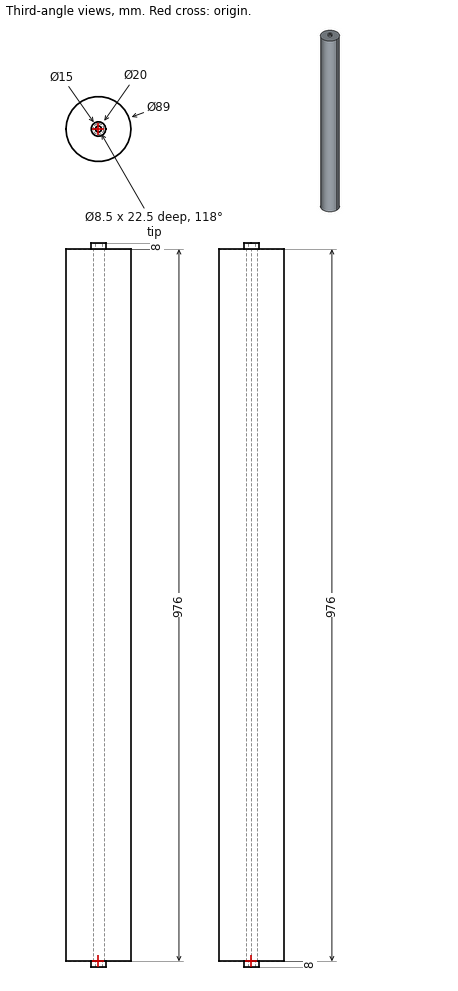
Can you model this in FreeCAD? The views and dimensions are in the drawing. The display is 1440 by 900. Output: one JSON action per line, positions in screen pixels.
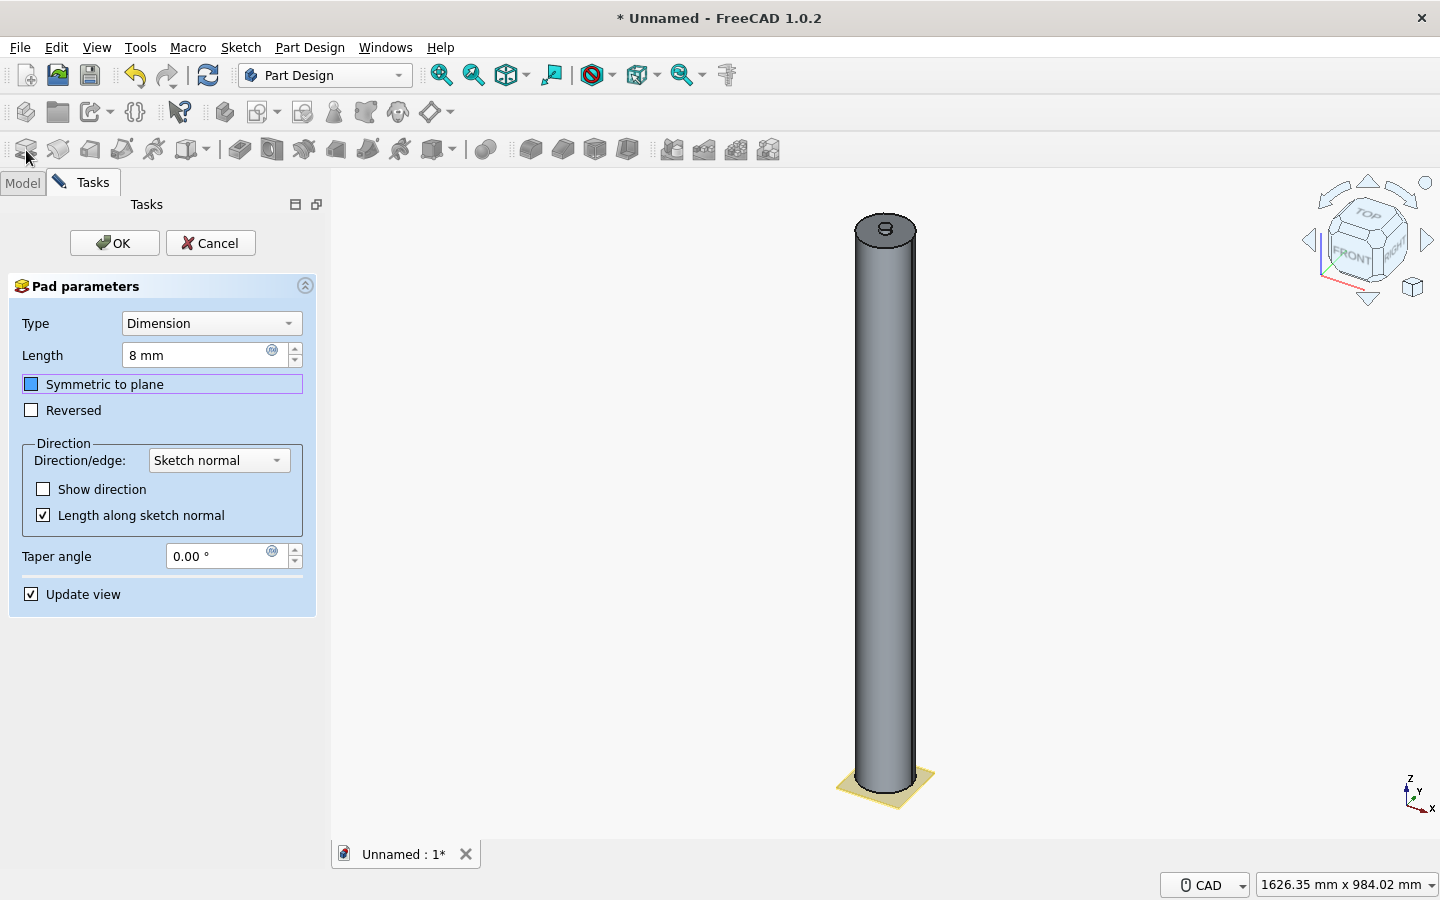
{"action": "left_click", "coordinate": [115, 243]}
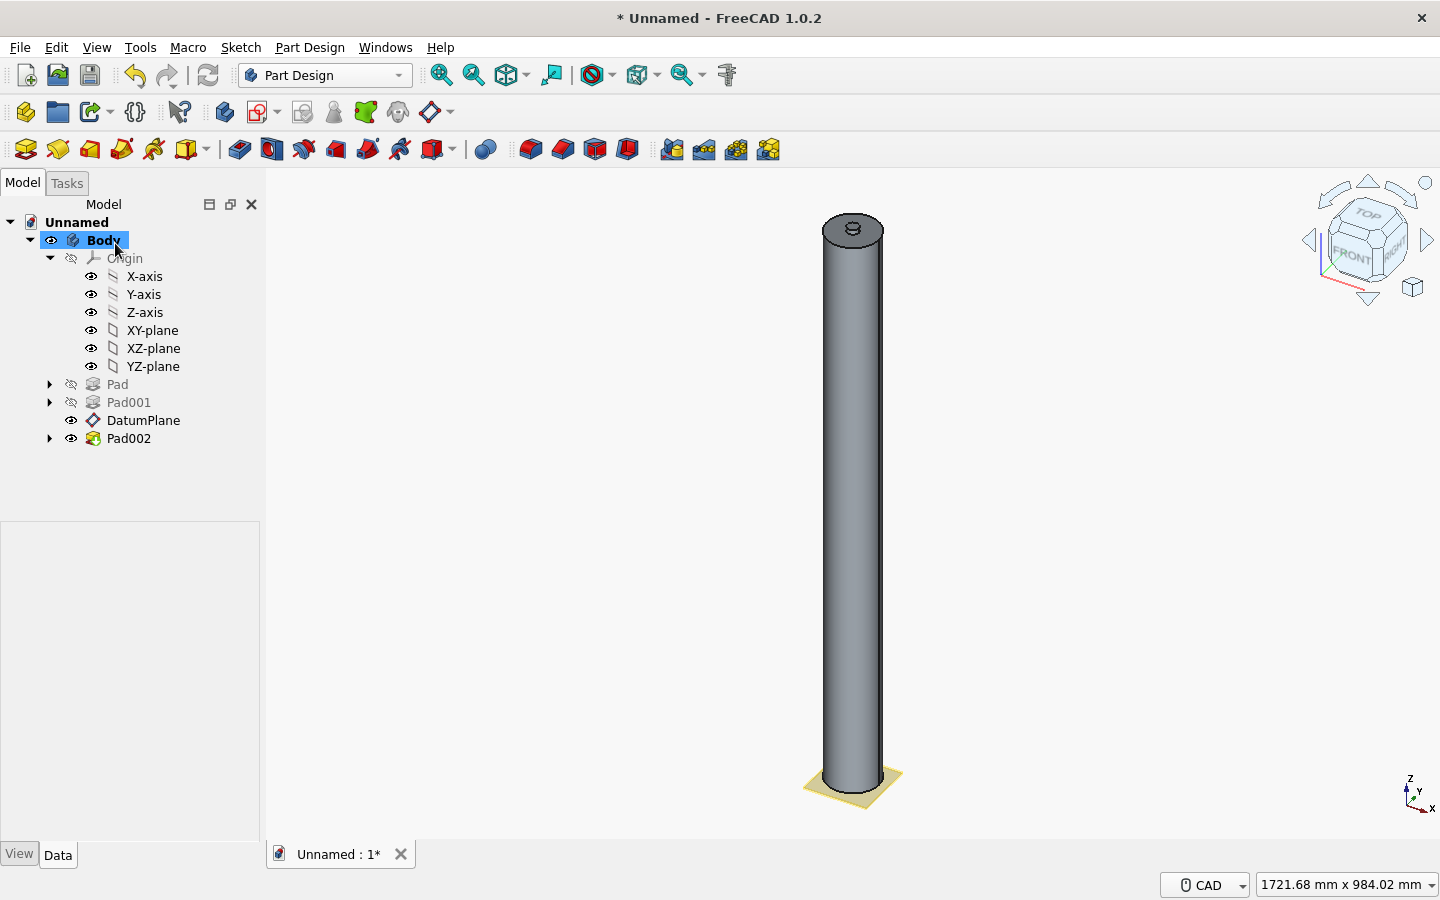
{"action": "left_click", "coordinate": [116, 420]}
{"action": "key", "text": "space"}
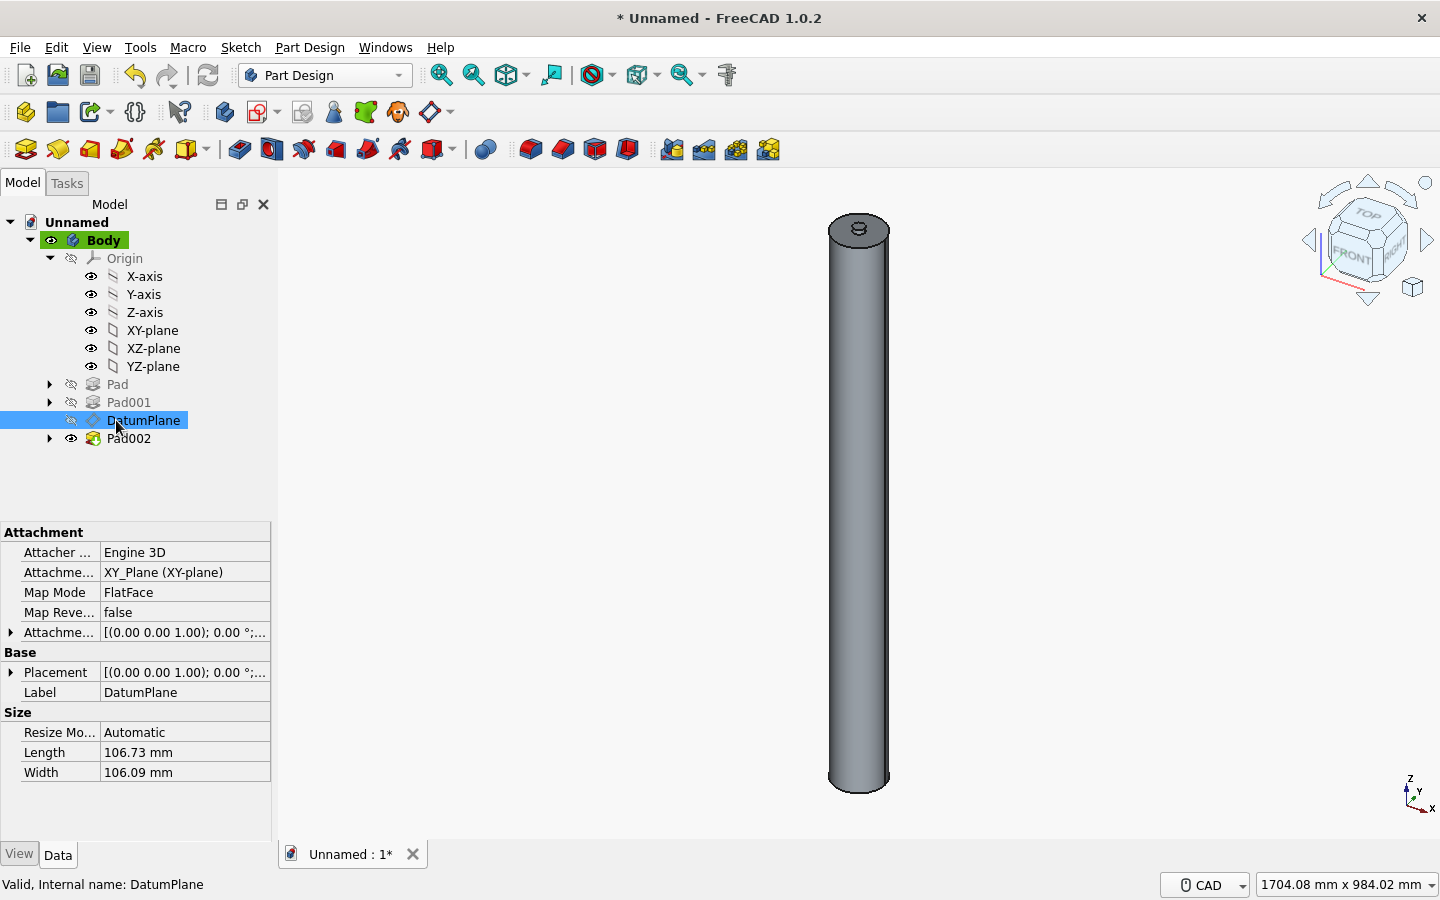
{"action": "key", "text": "5"}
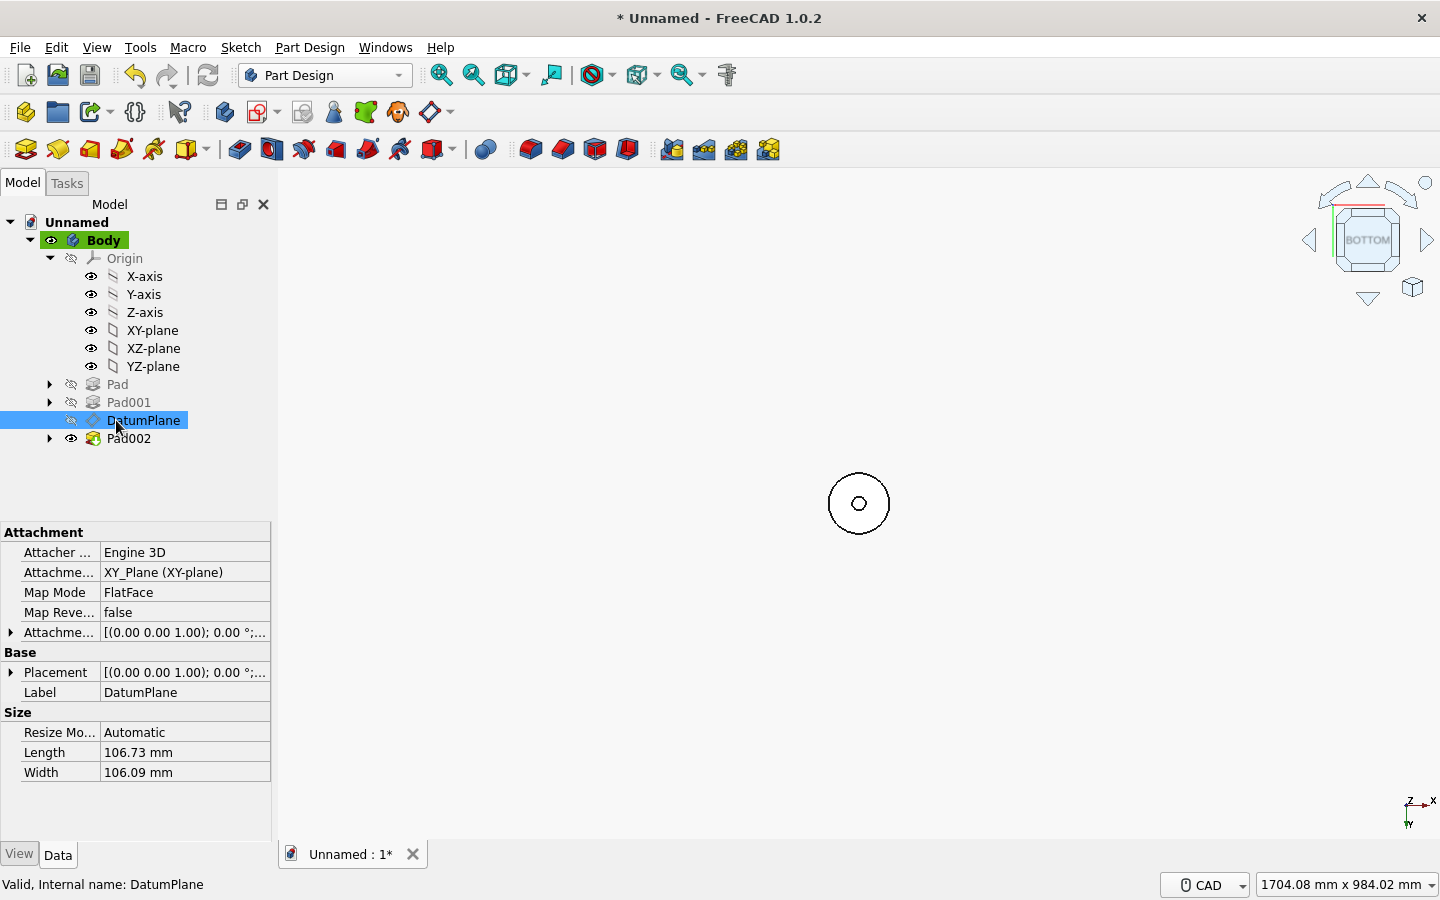
{"action": "left_click", "coordinate": [442, 76]}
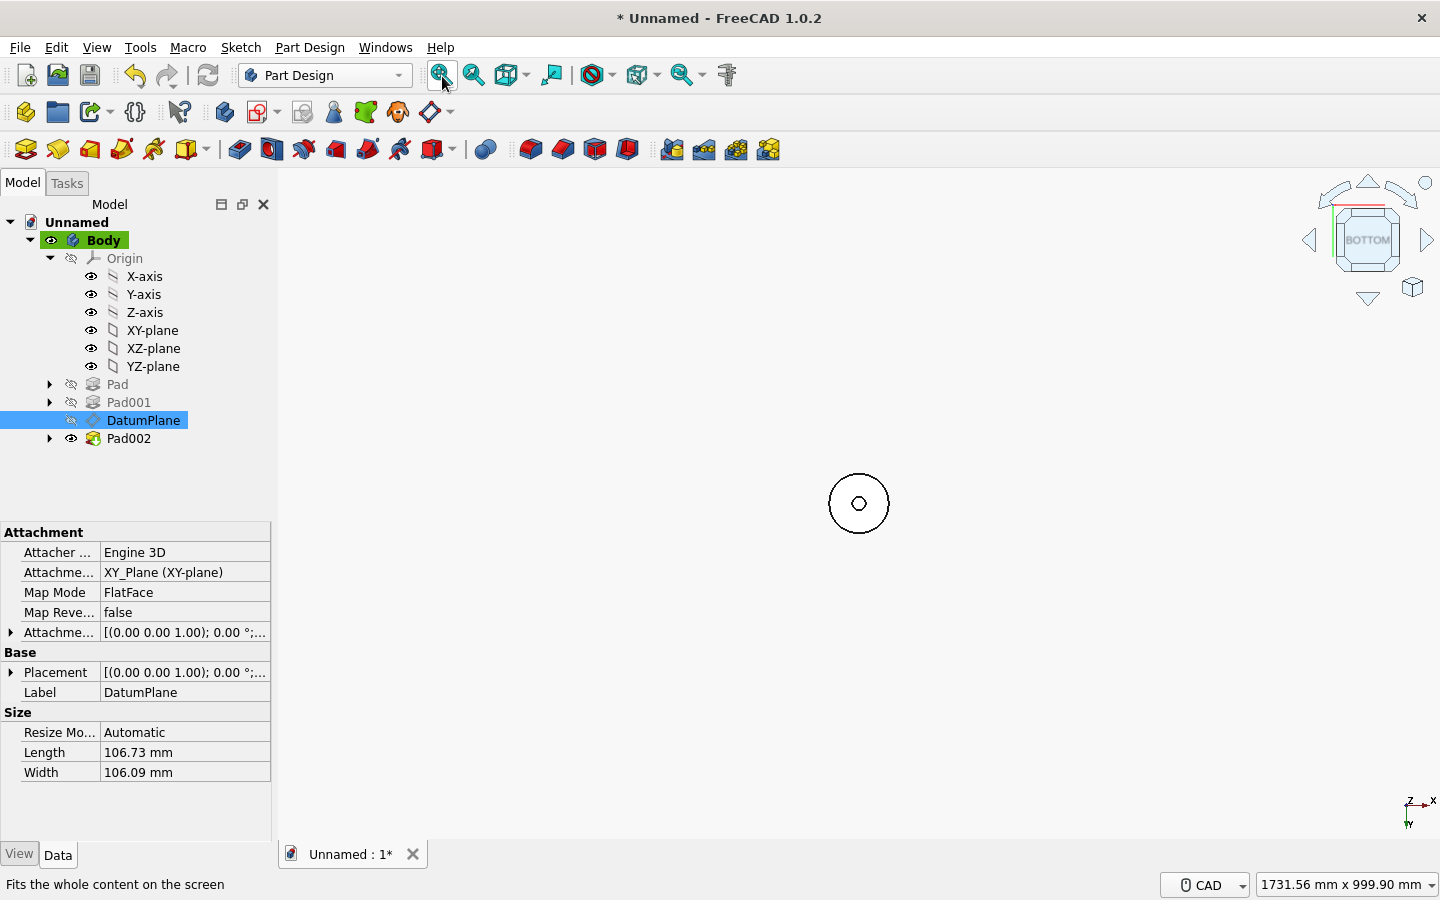
{"action": "scroll", "coordinate": [859, 502], "scroll_direction": "up", "scroll_amount": 3}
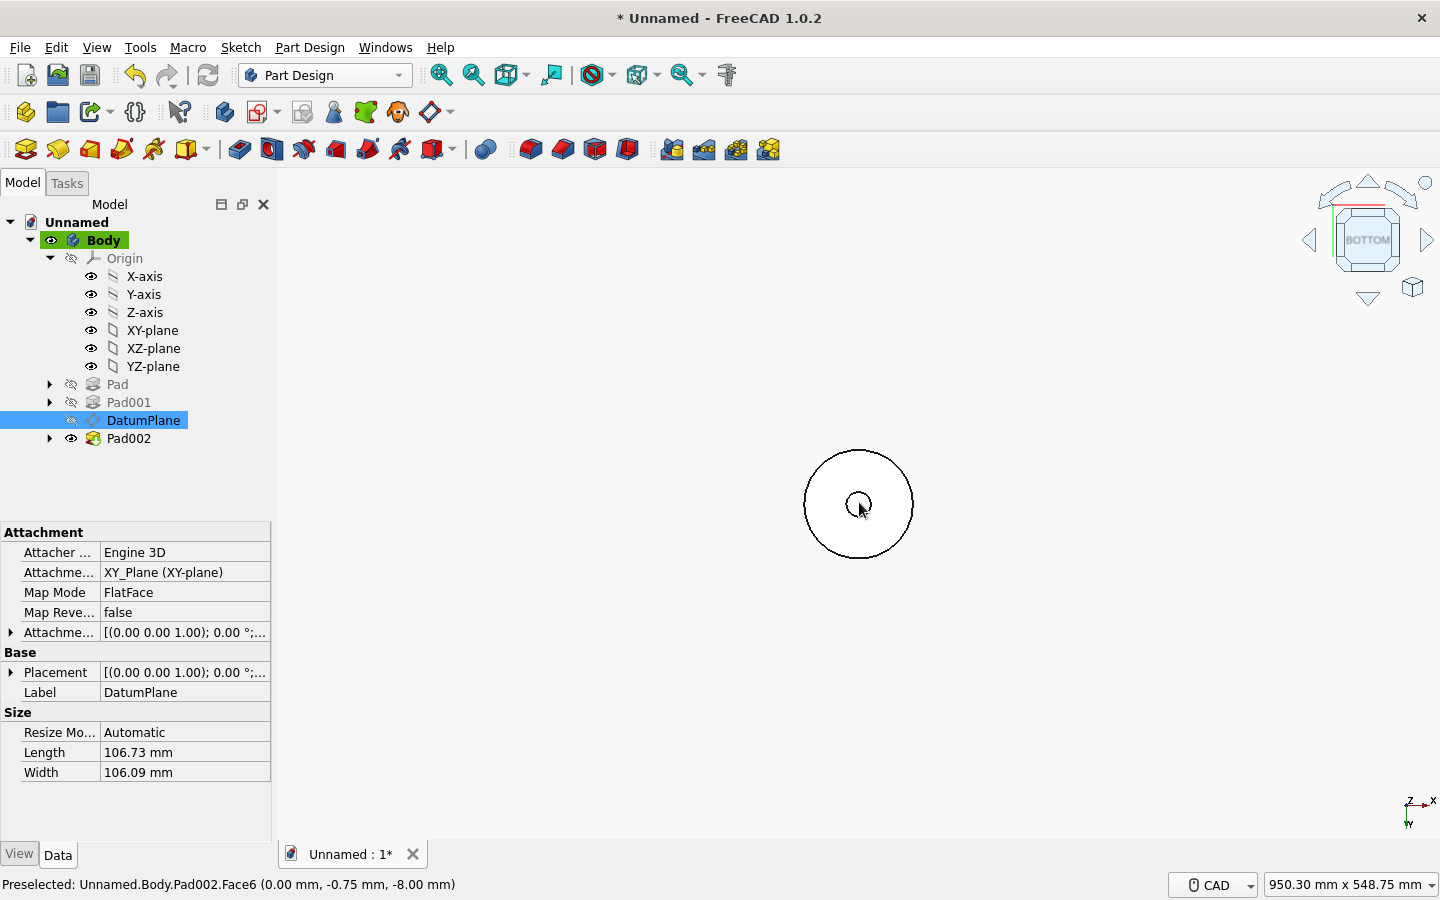
{"action": "left_click", "coordinate": [859, 503]}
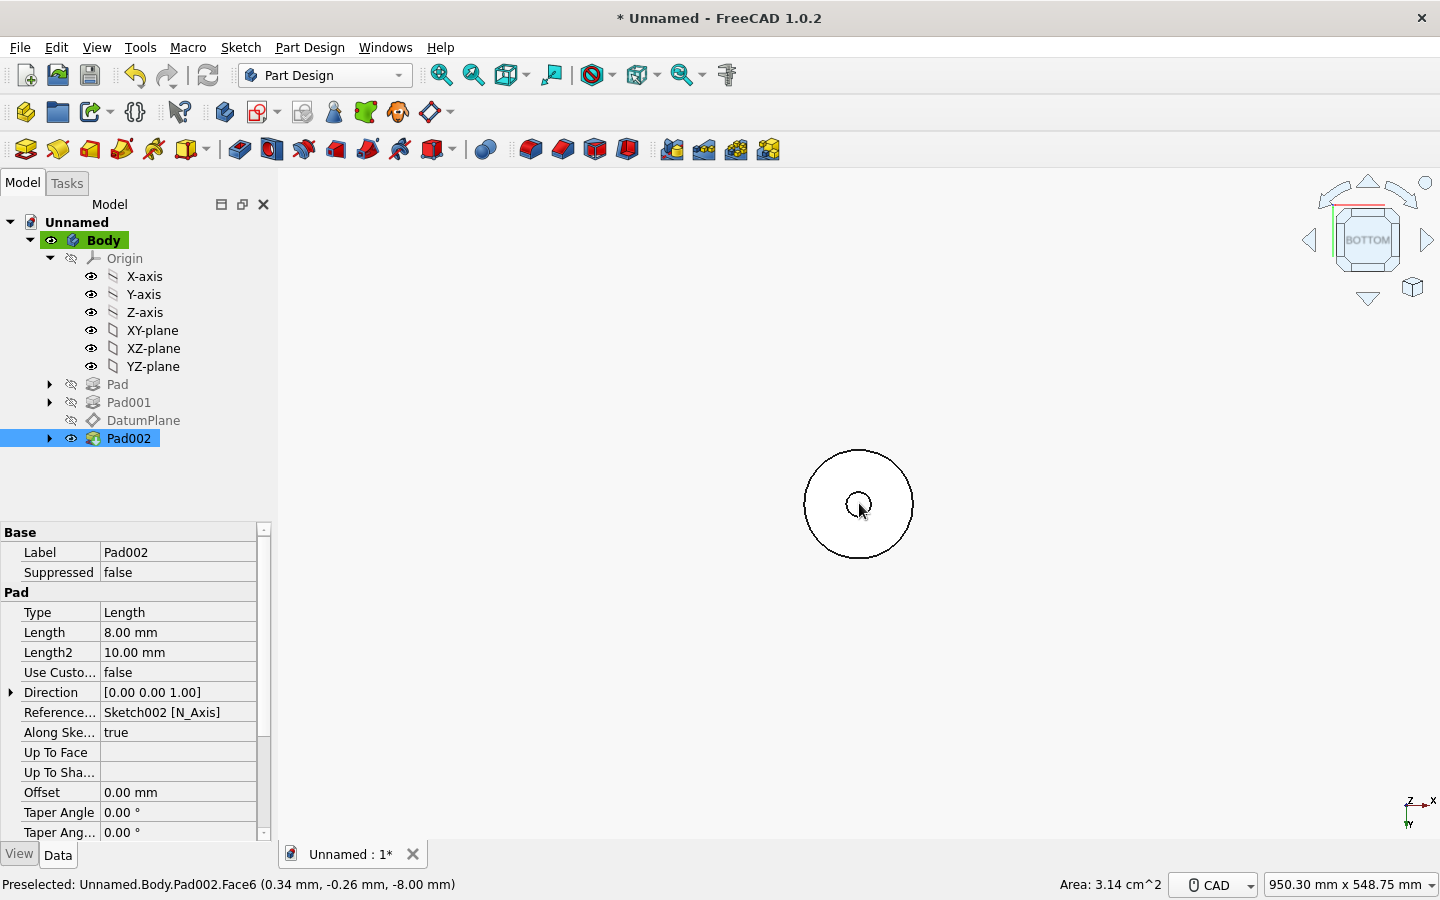
{"action": "left_click", "coordinate": [258, 112]}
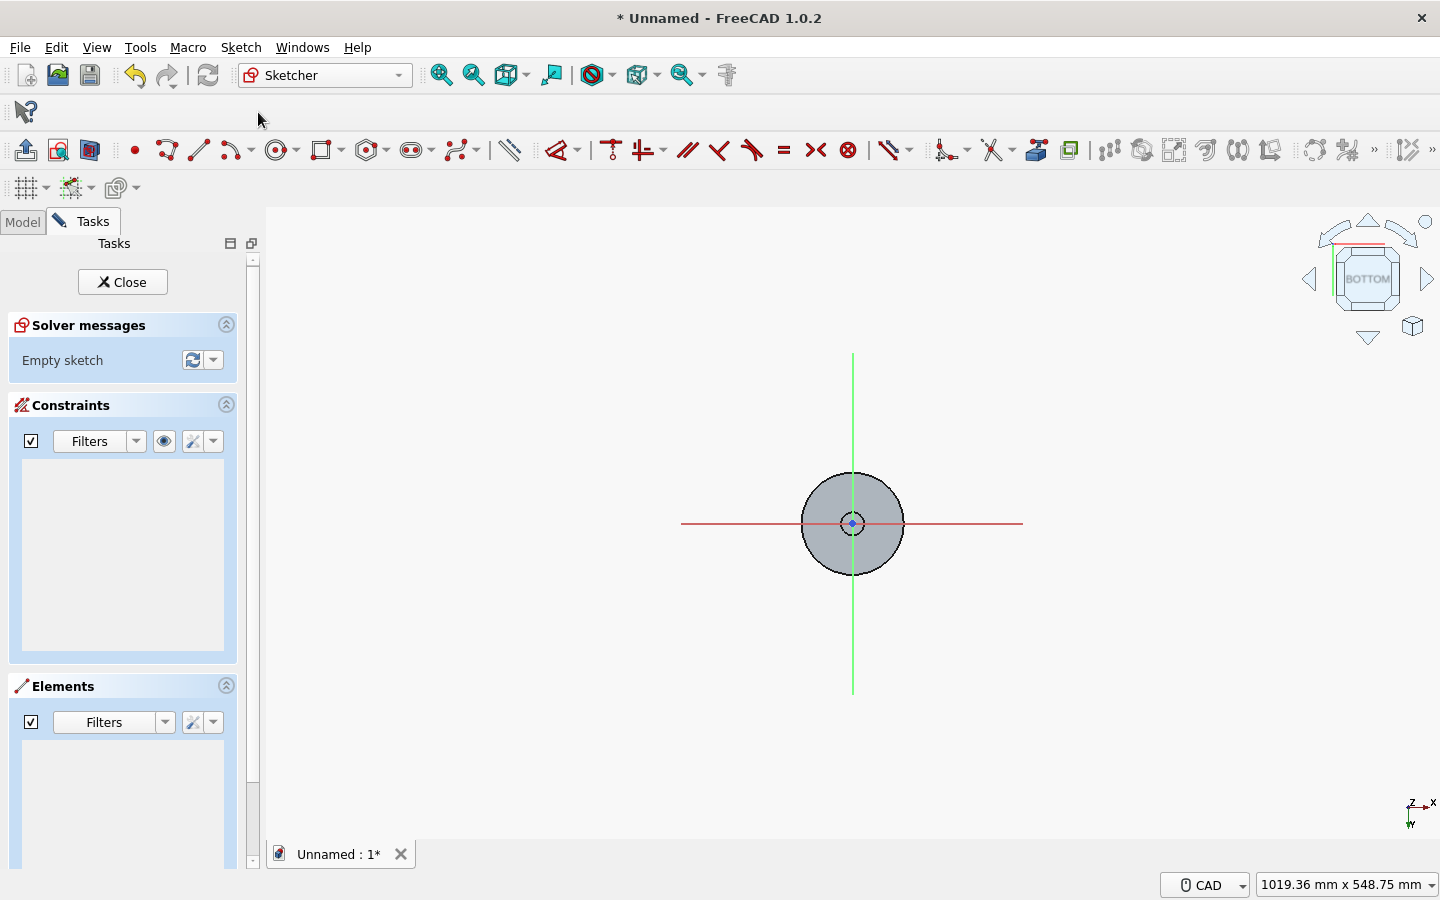
{"action": "scroll", "coordinate": [856, 524], "scroll_direction": "up", "scroll_amount": 15}